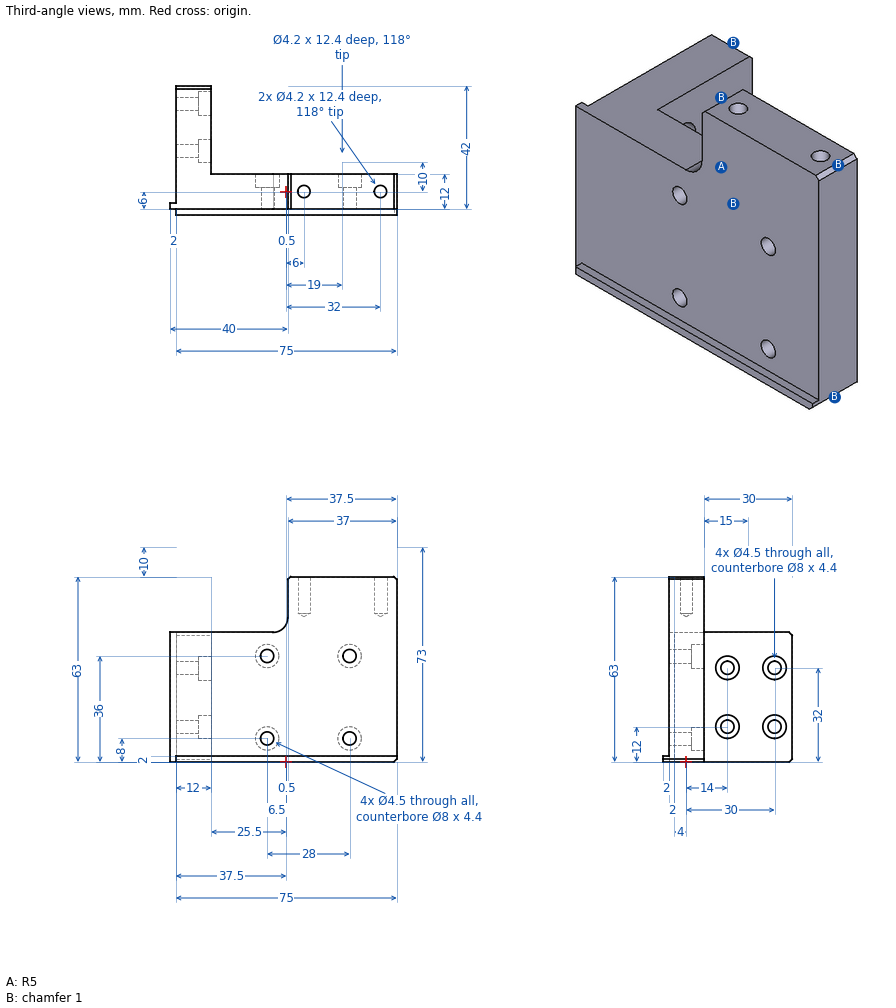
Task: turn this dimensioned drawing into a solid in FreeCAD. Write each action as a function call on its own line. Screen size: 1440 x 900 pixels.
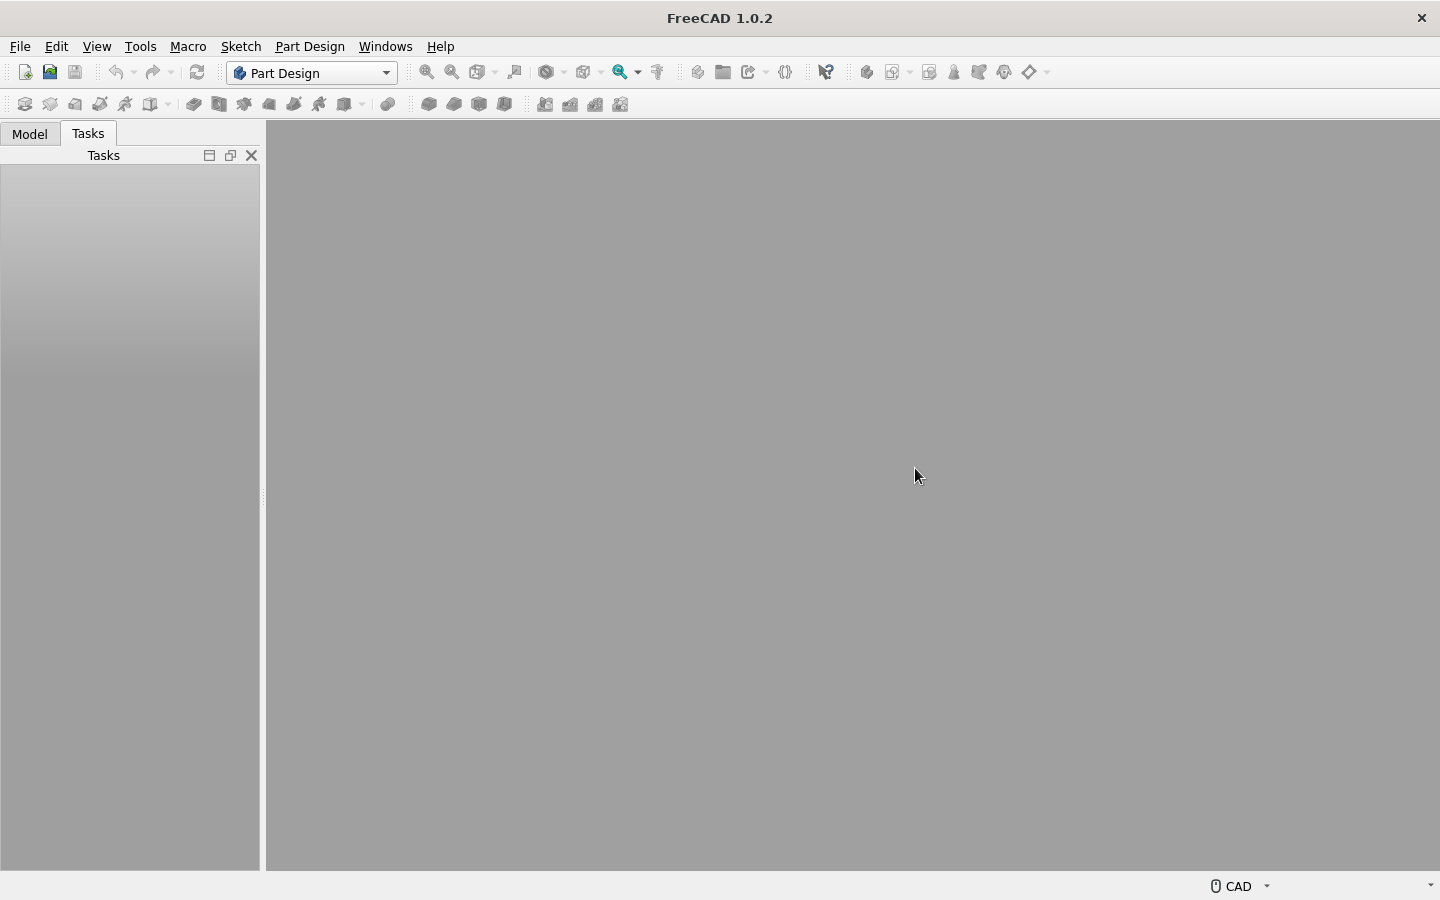
click(25, 72)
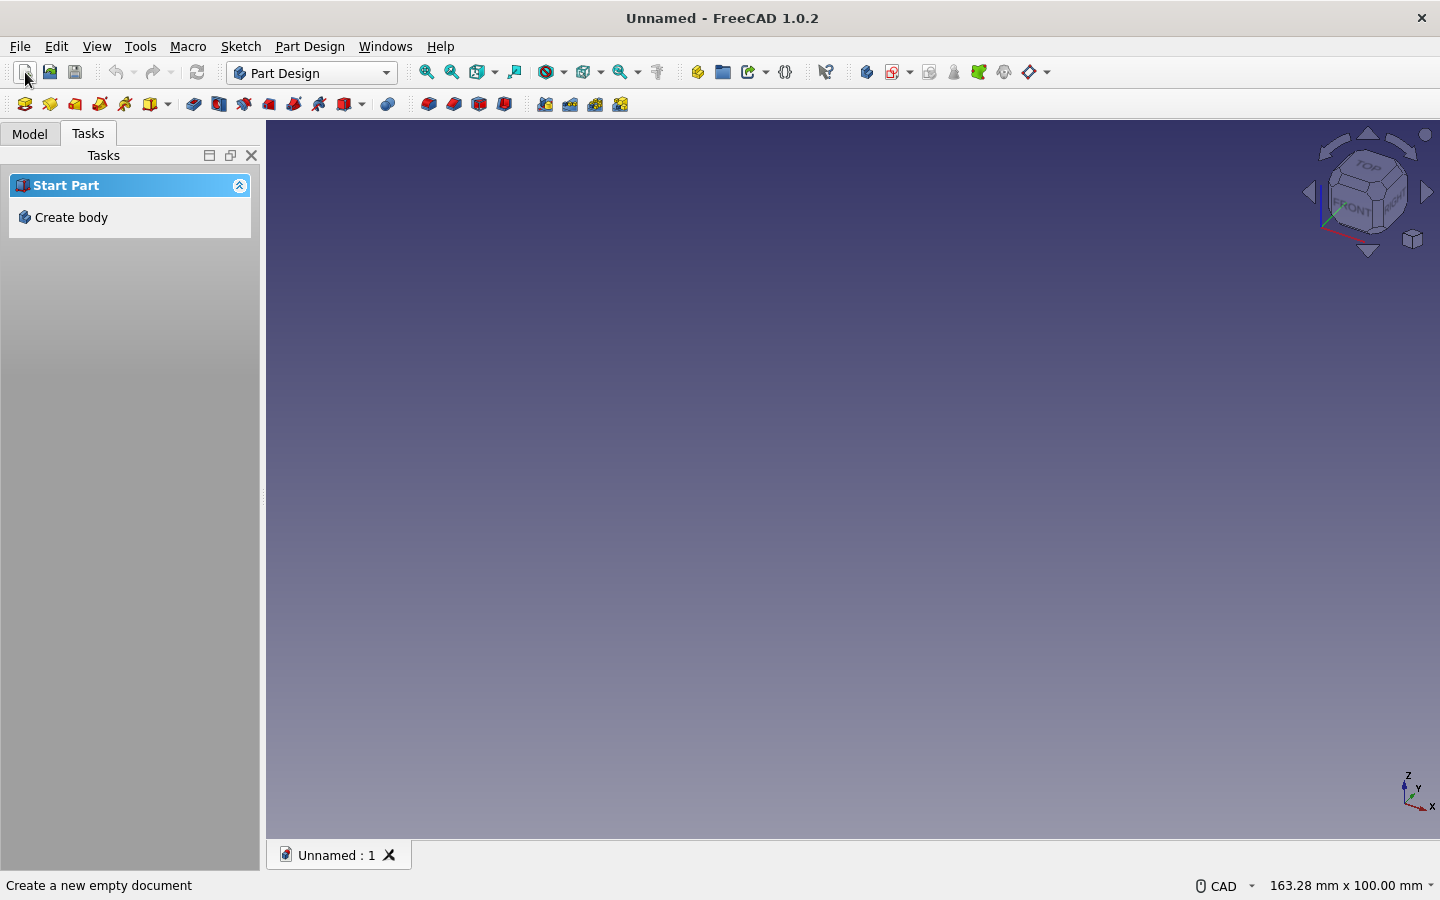
click(892, 72)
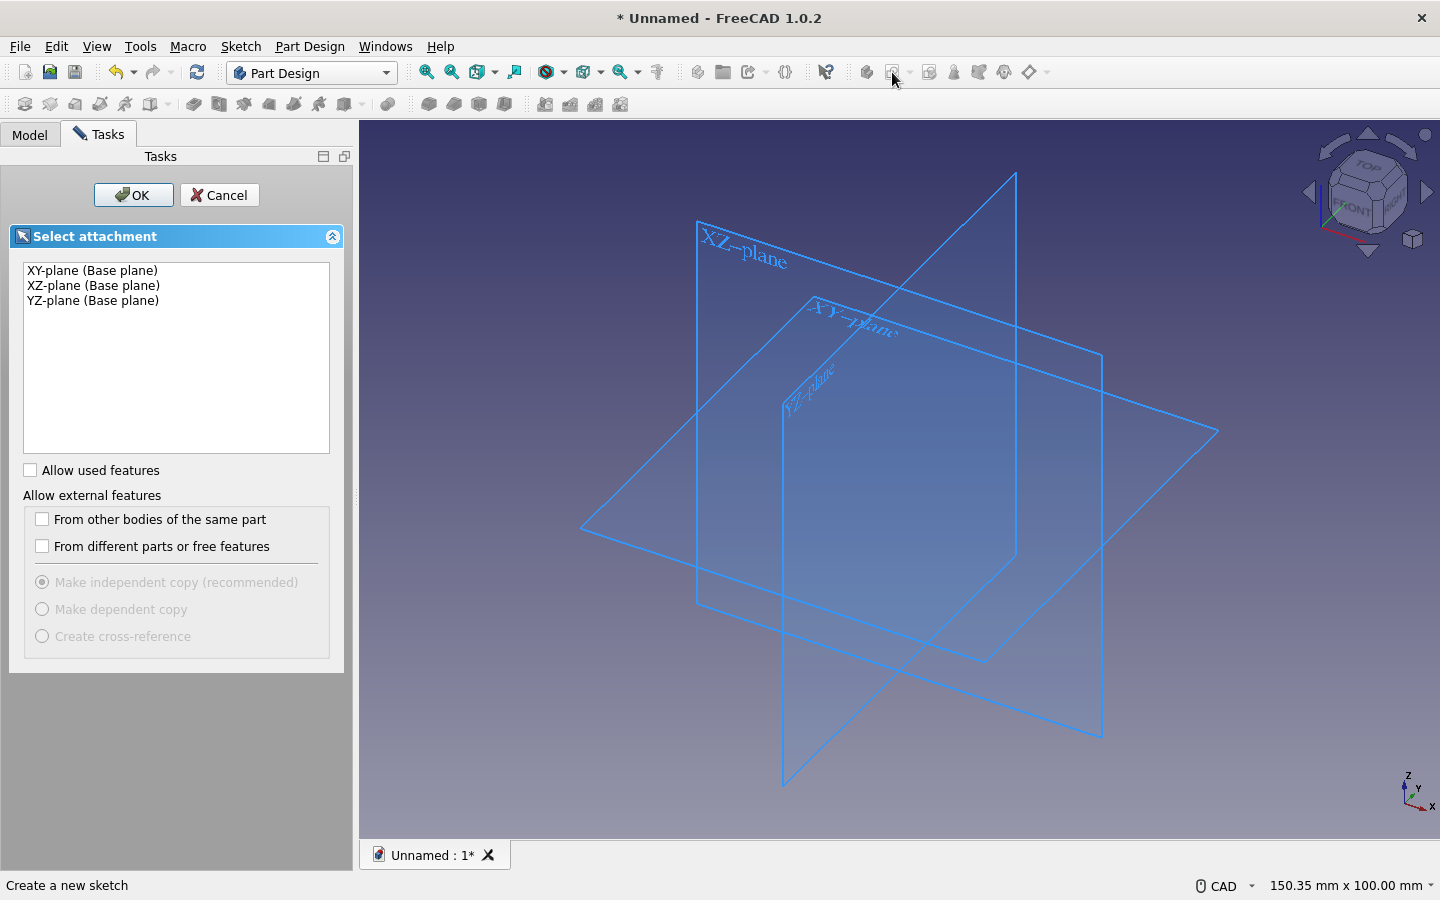
click(84, 270)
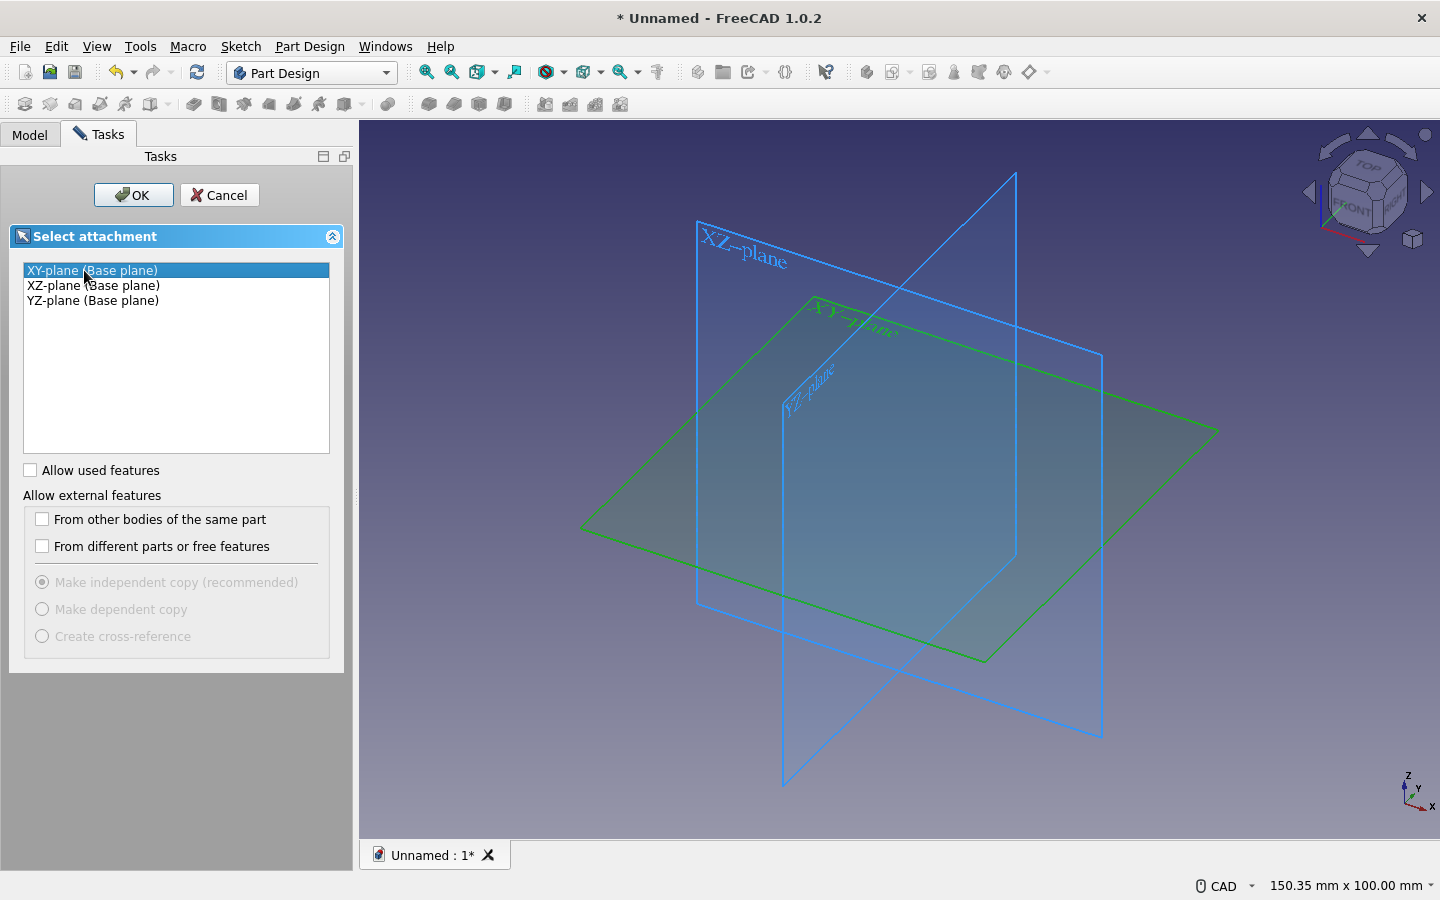
click(134, 195)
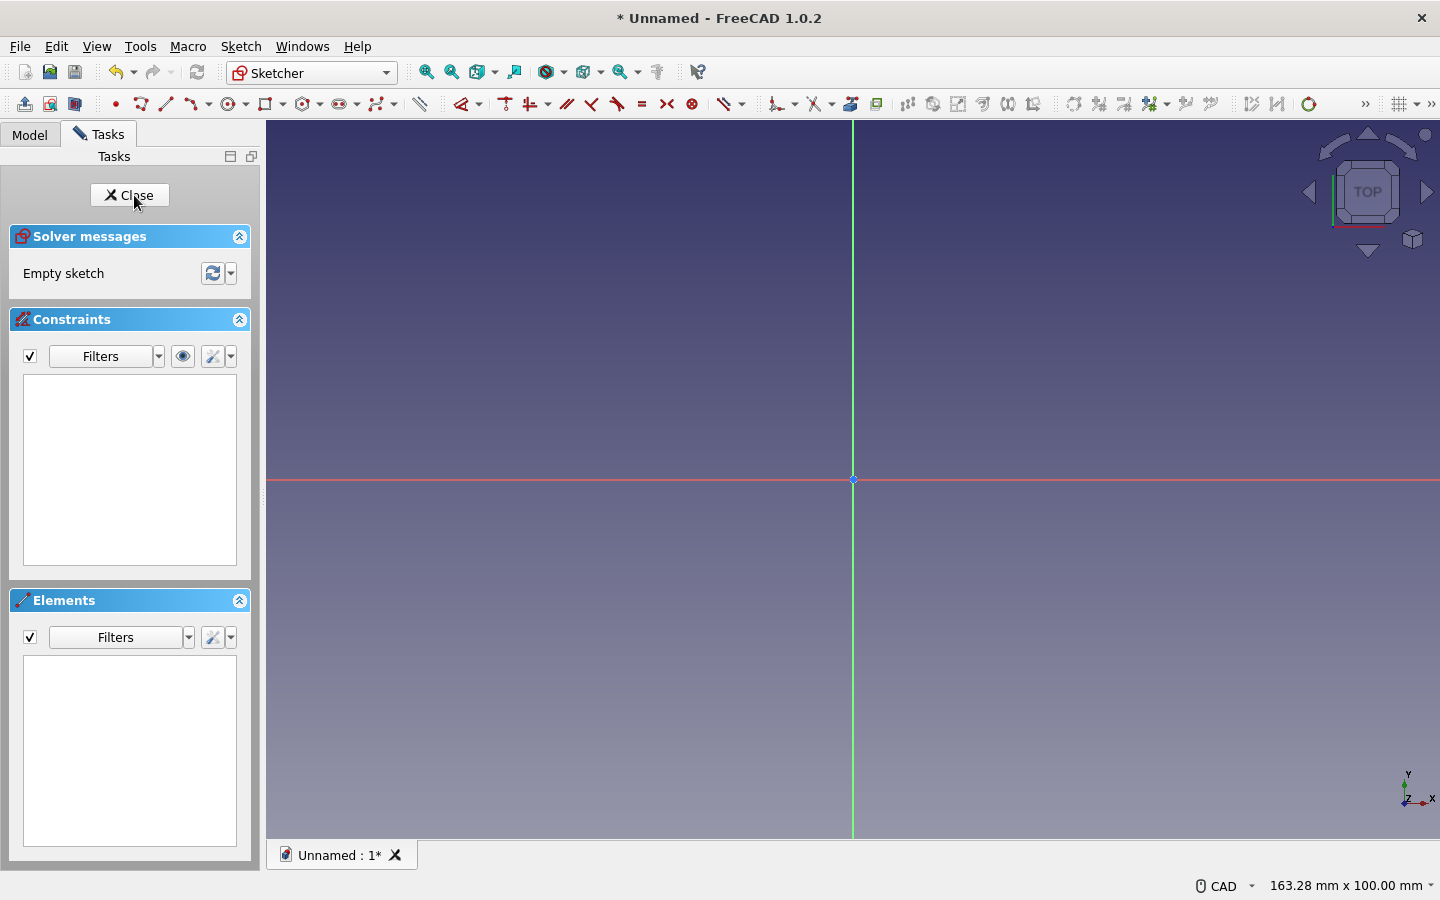
key(g)
key(v)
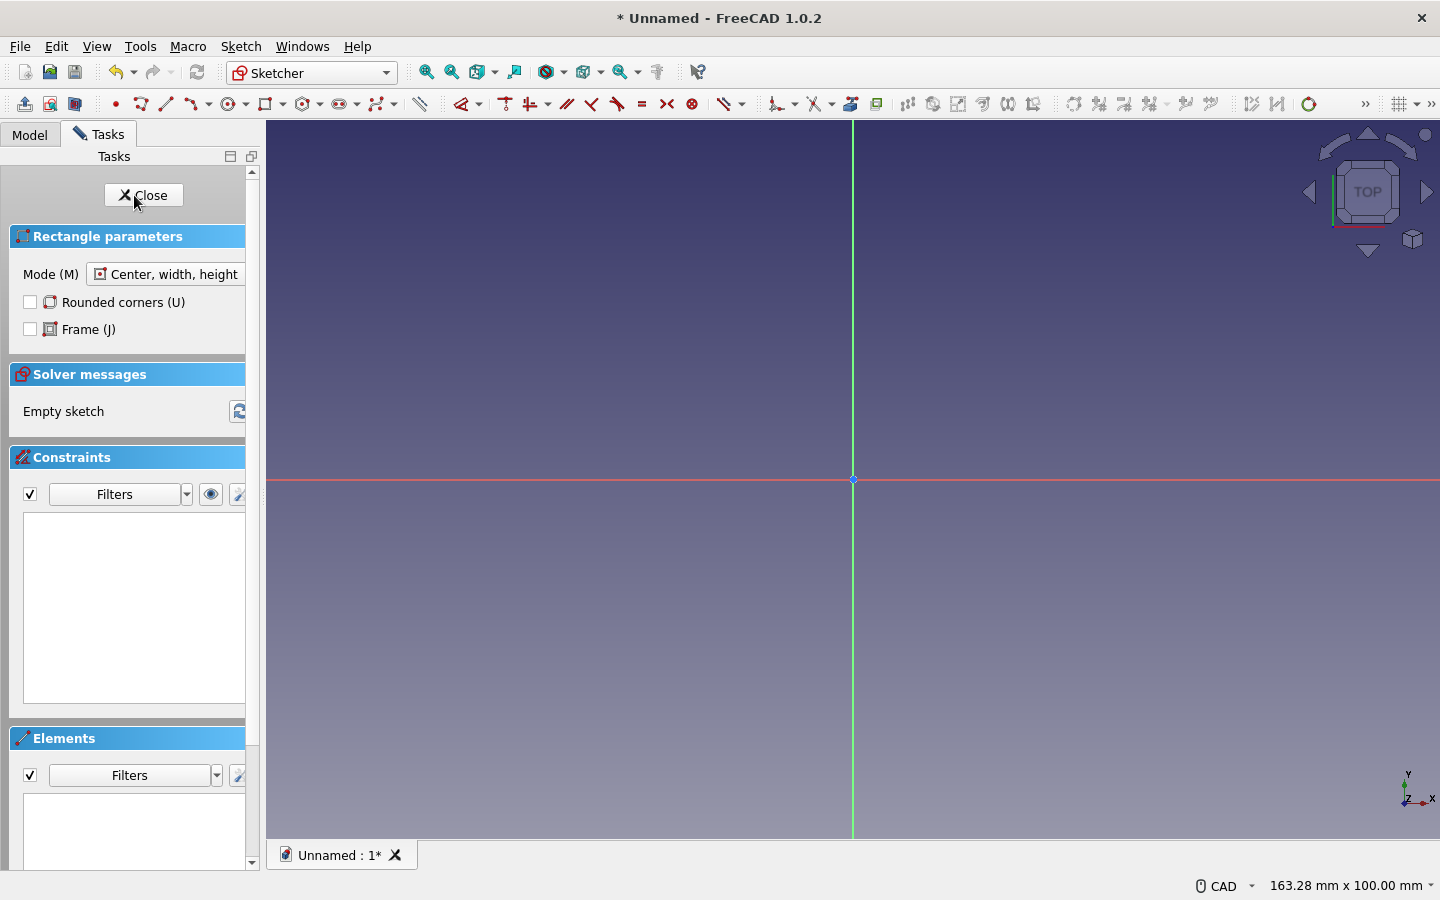
click(853, 480)
move(1123, 436)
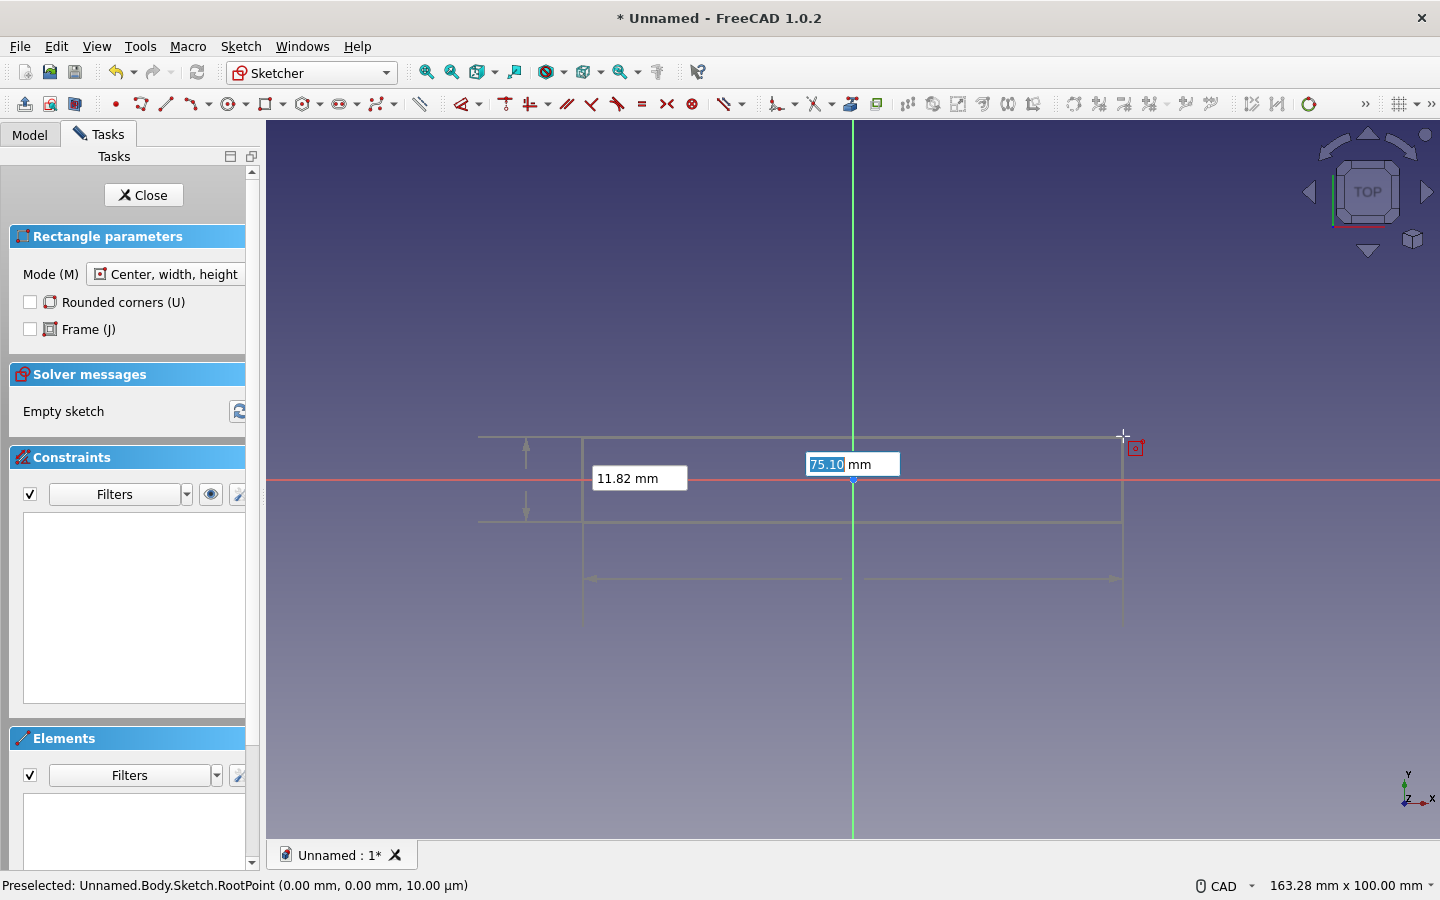
text(75)
key(Tab)
text(12)
key(Return)
key(Escape)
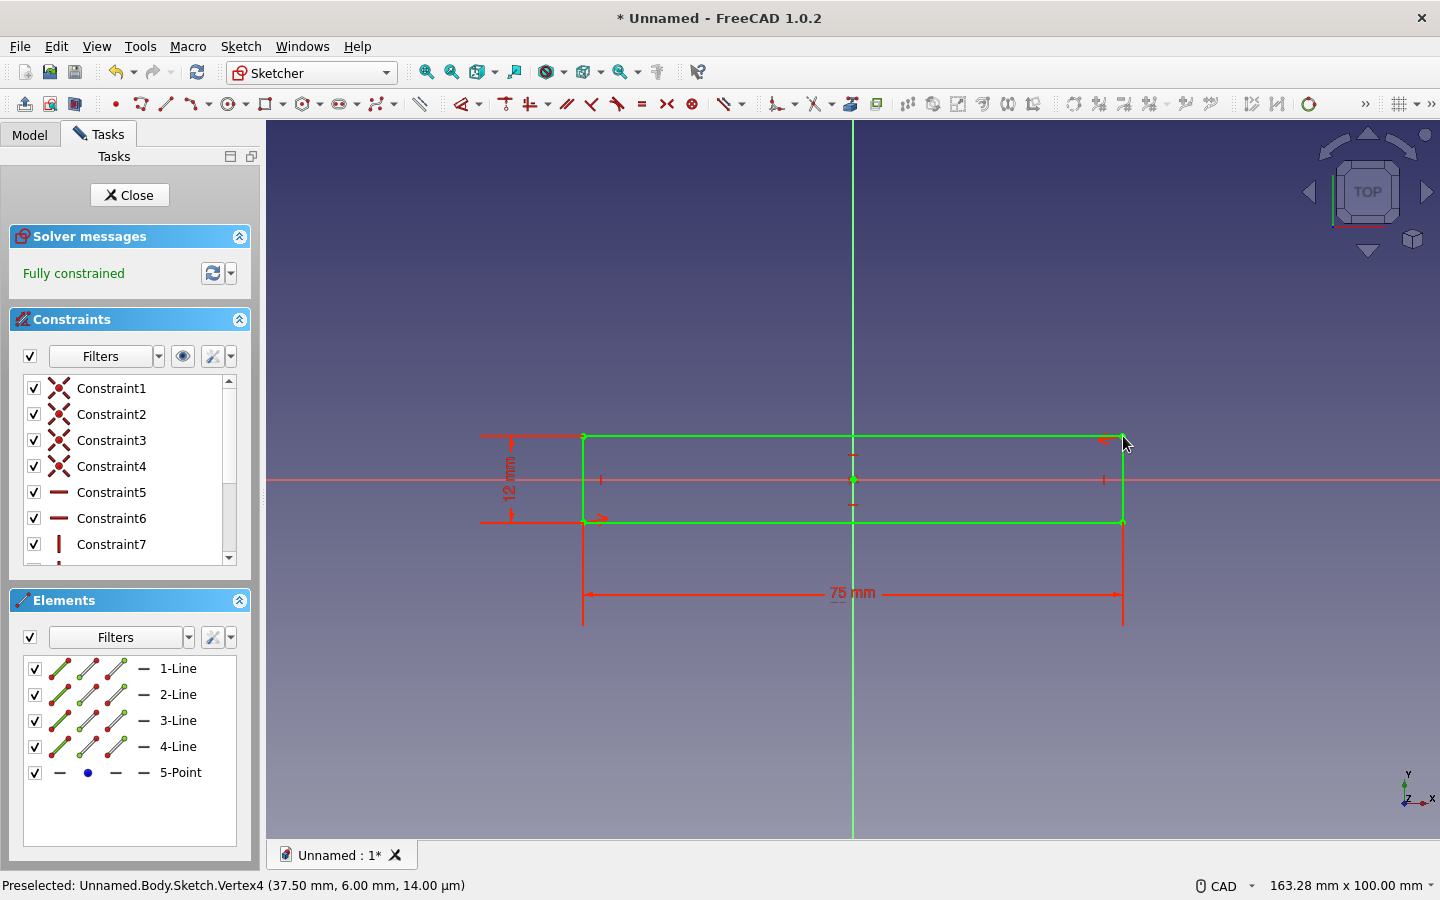
click(130, 195)